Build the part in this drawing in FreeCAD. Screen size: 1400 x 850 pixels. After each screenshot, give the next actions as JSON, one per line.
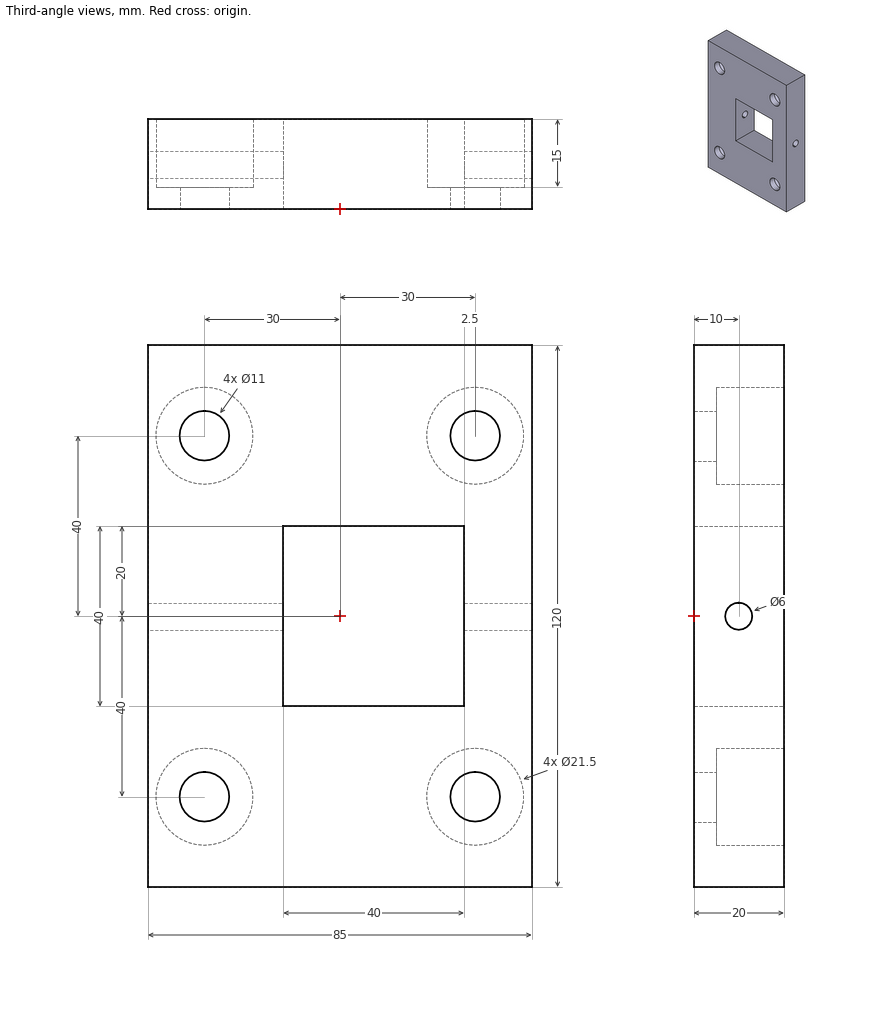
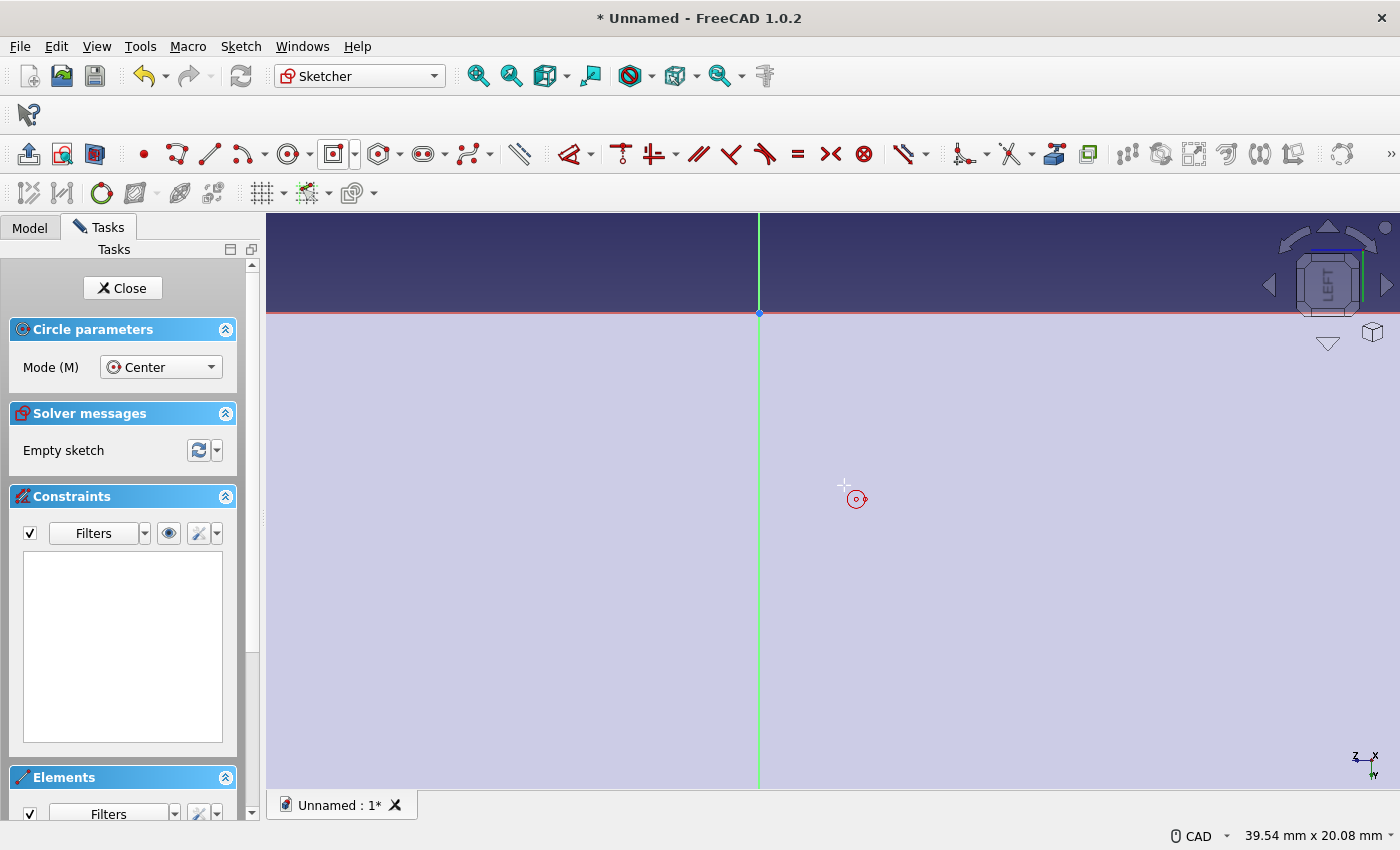
{"action": "left_click", "coordinate": [759, 600]}
{"action": "left_click", "coordinate": [820, 539]}
{"action": "key", "text": "Escape"}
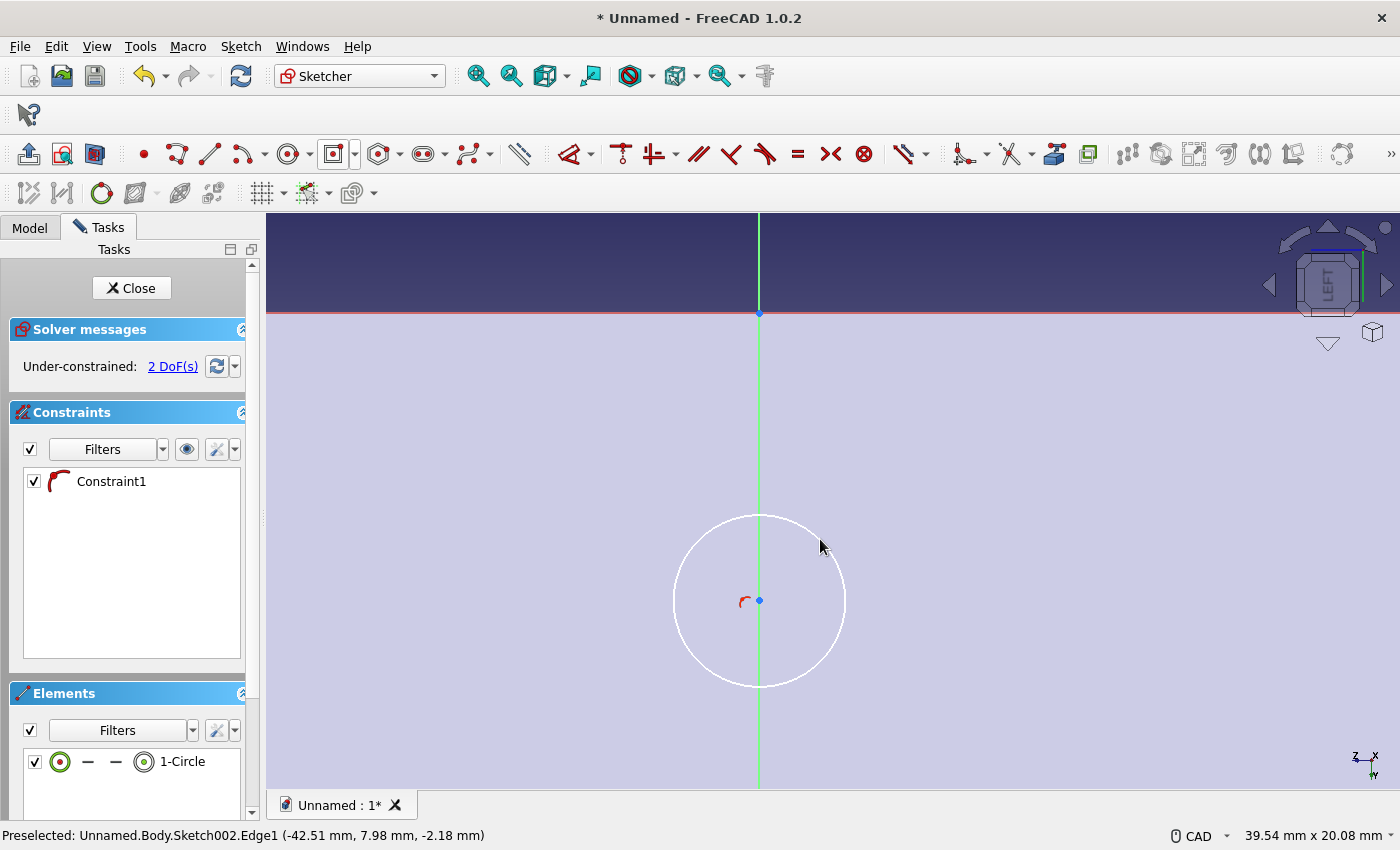
{"action": "key", "text": "d"}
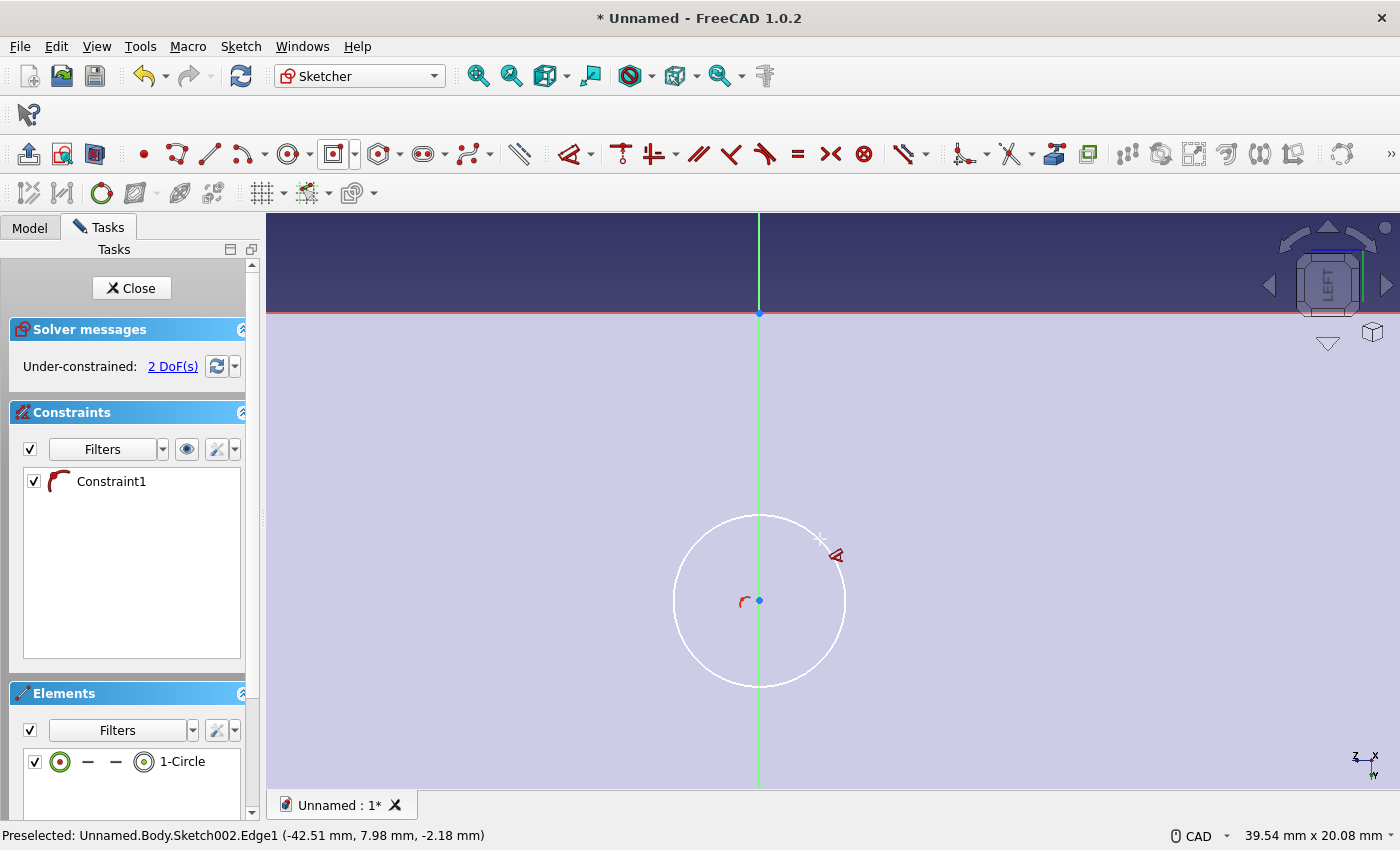
{"action": "left_click", "coordinate": [820, 540]}
{"action": "left_click", "coordinate": [843, 517]}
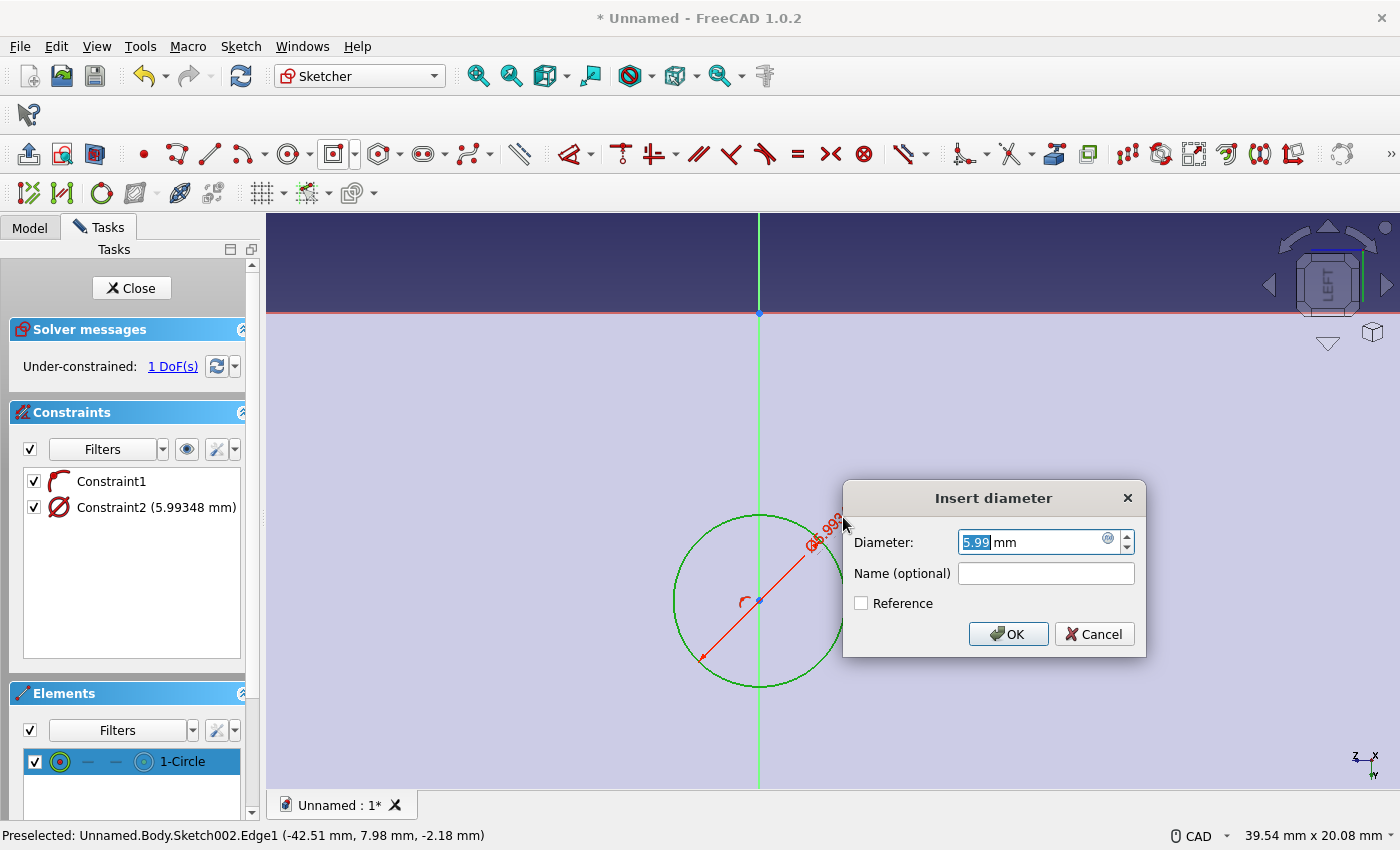
{"action": "type", "text": "6"}
{"action": "key", "text": "Return"}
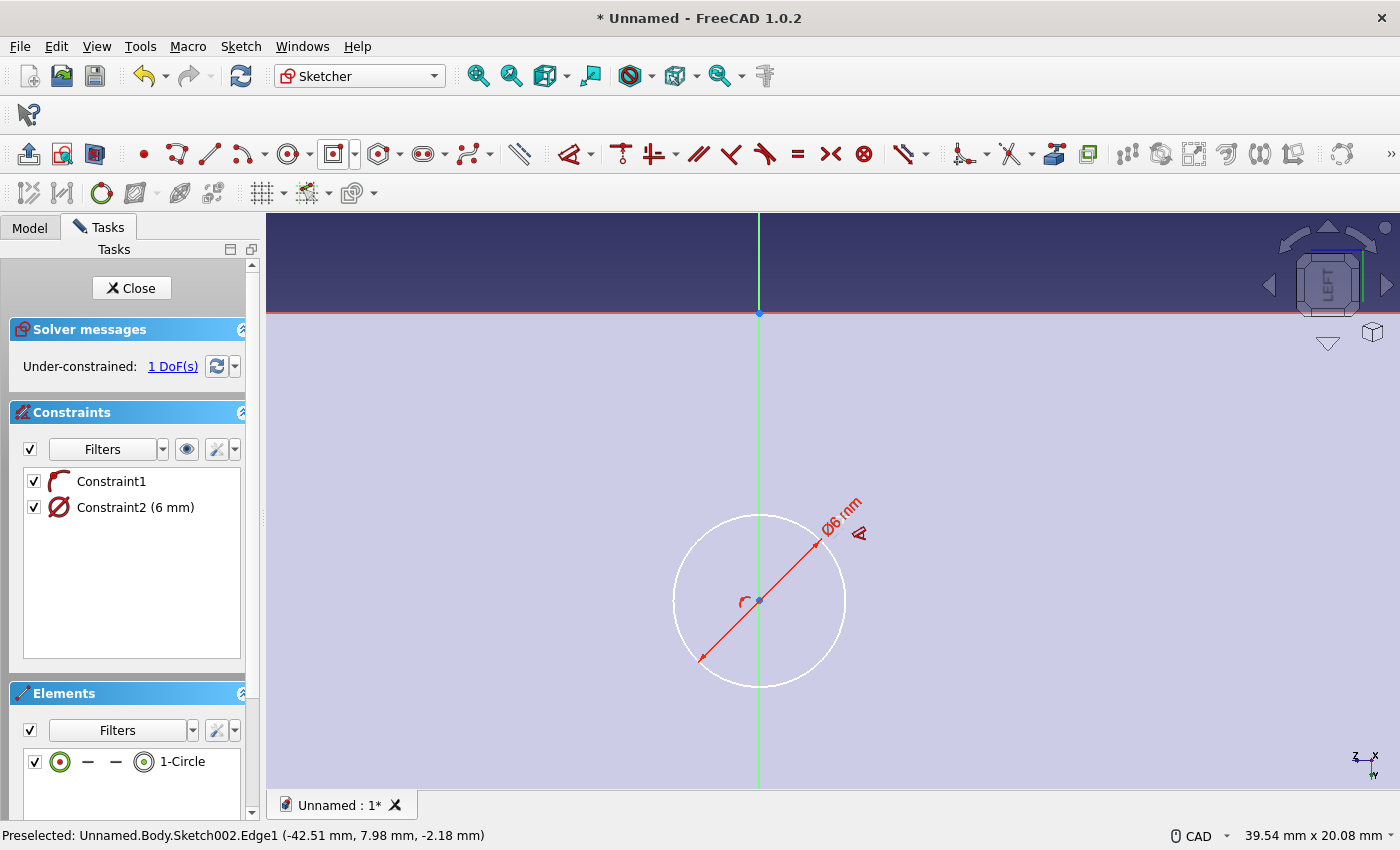
{"action": "left_click", "coordinate": [759, 601]}
{"action": "left_click", "coordinate": [793, 457]}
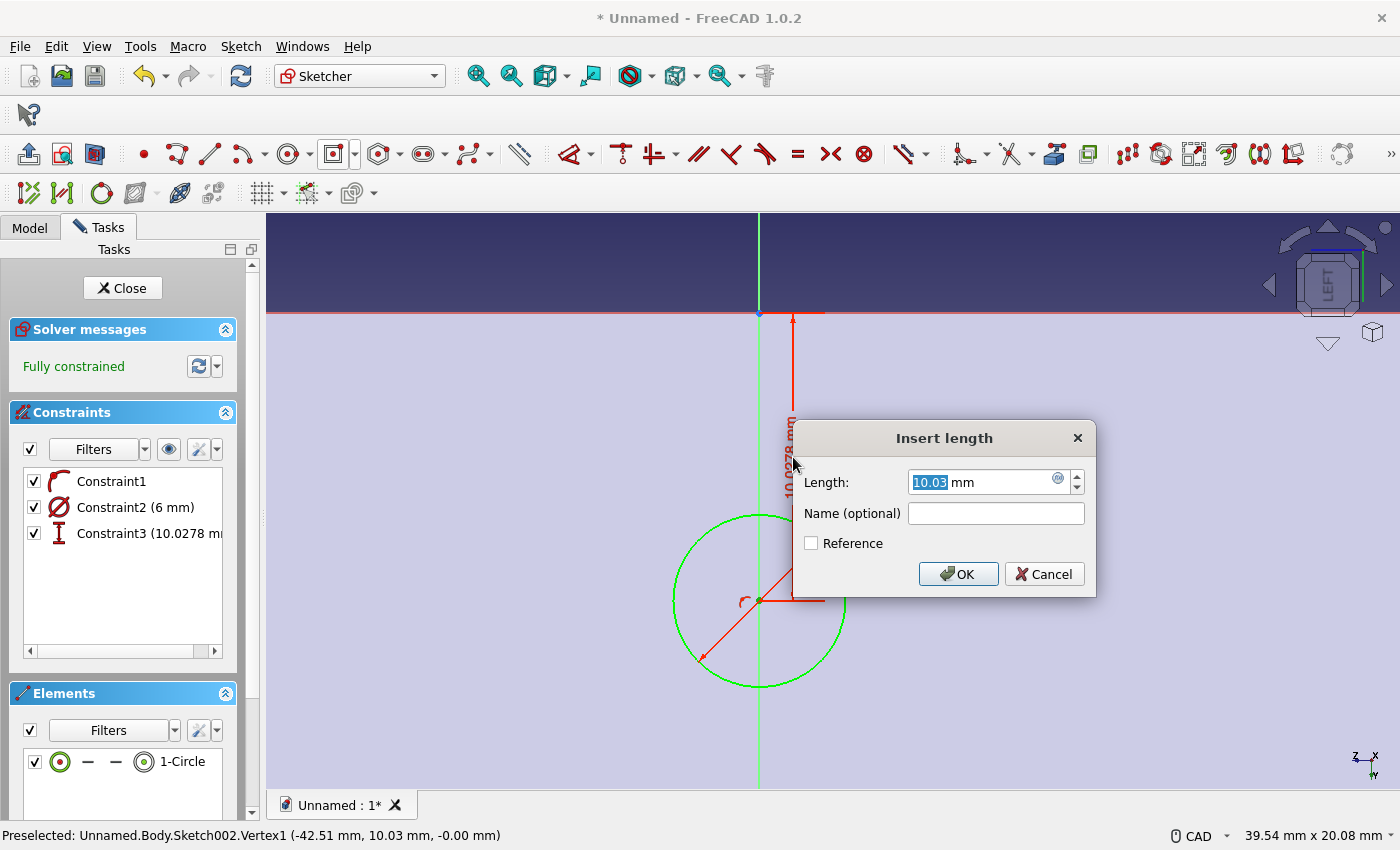
{"action": "type", "text": "10"}
{"action": "key", "text": "Return"}
{"action": "key", "text": "Escape"}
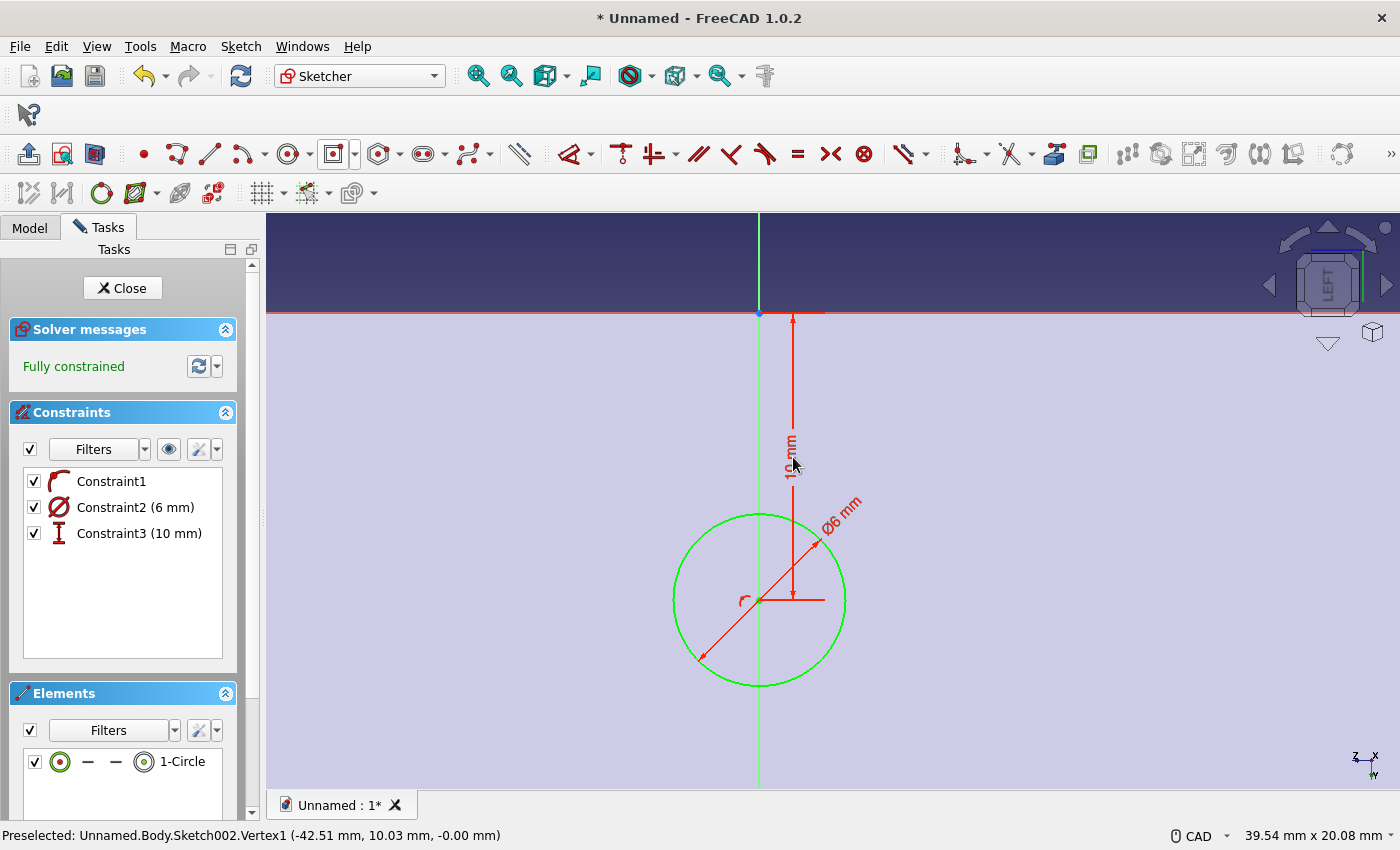
{"action": "left_click", "coordinate": [123, 288]}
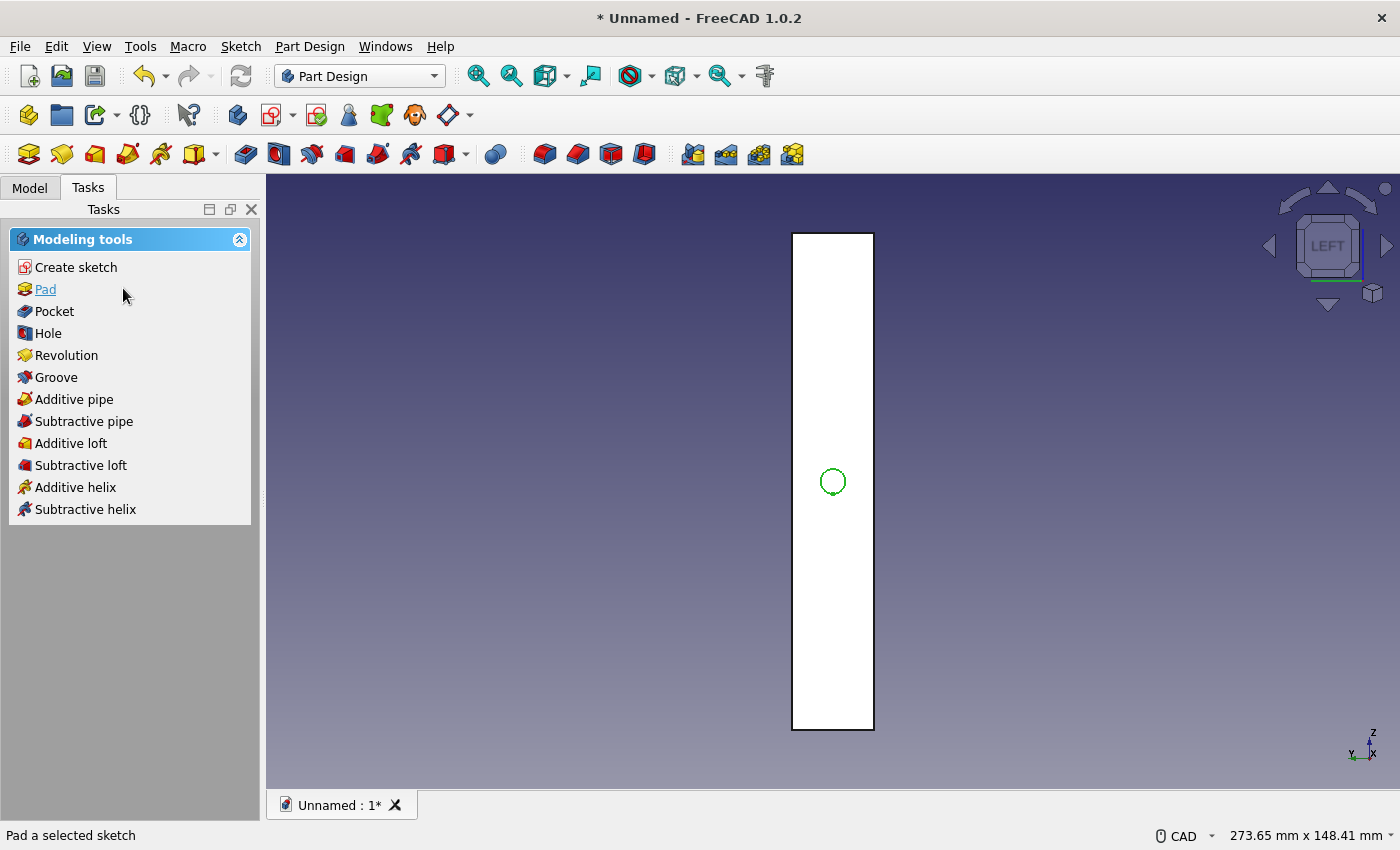
{"action": "left_click", "coordinate": [246, 154]}